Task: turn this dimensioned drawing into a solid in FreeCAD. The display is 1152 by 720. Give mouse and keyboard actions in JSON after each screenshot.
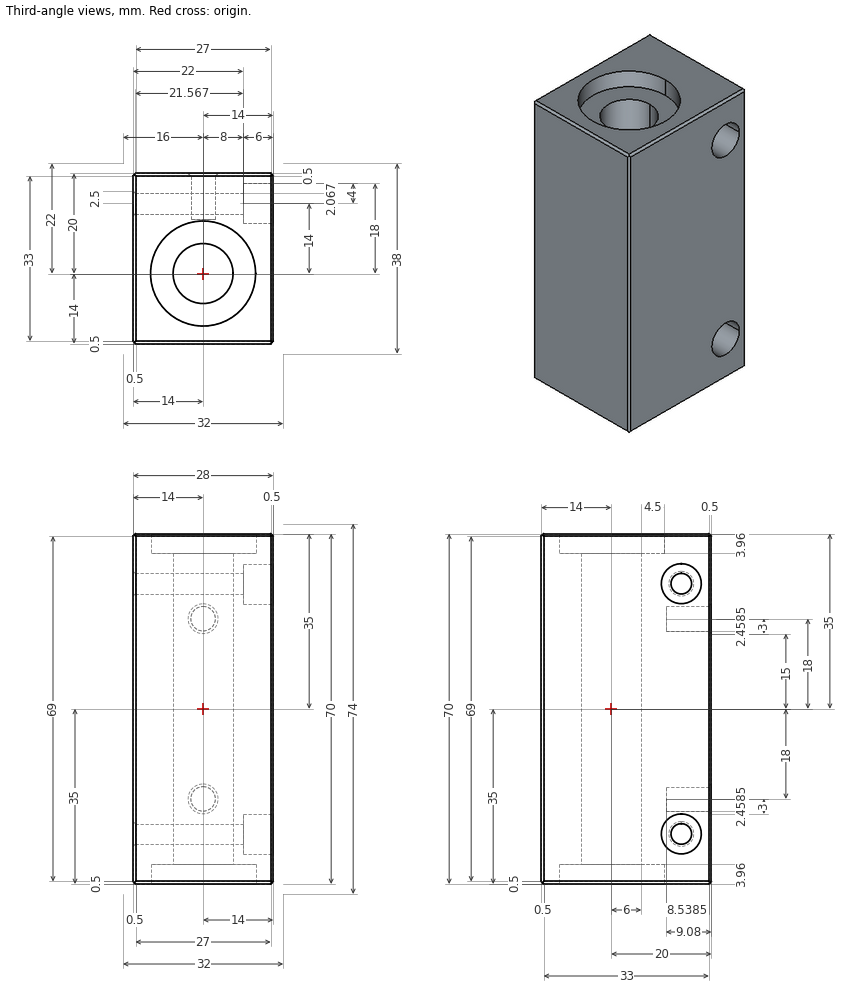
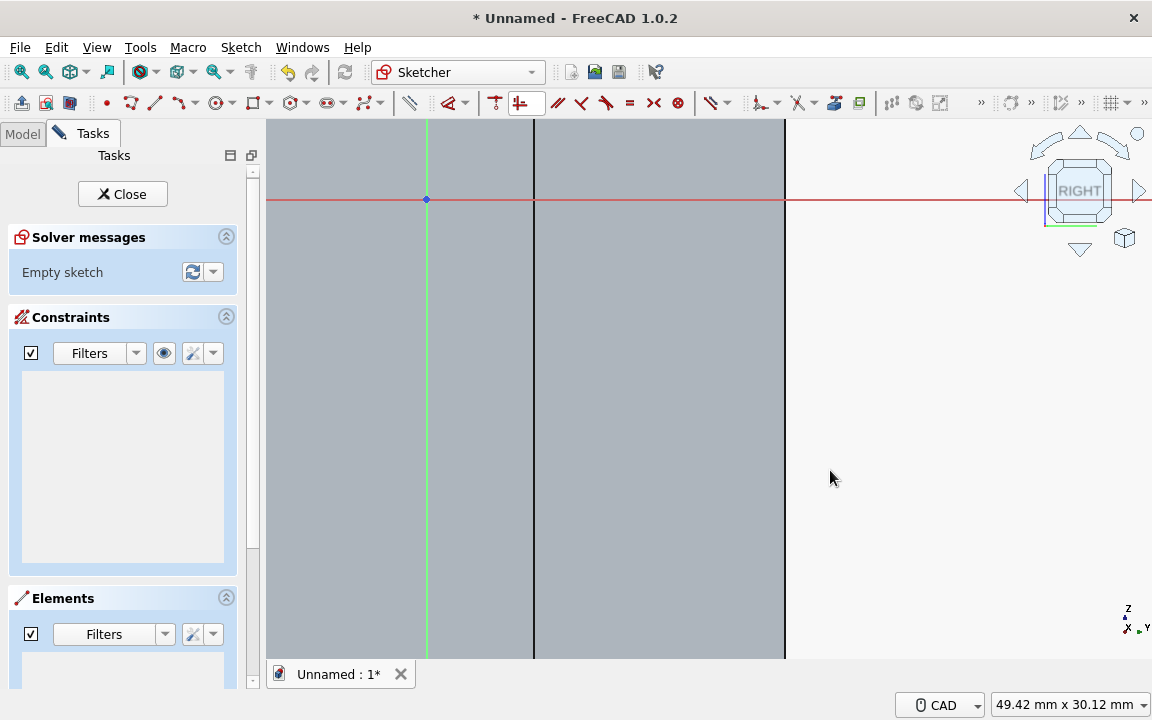
{"action": "left_click", "coordinate": [132, 104]}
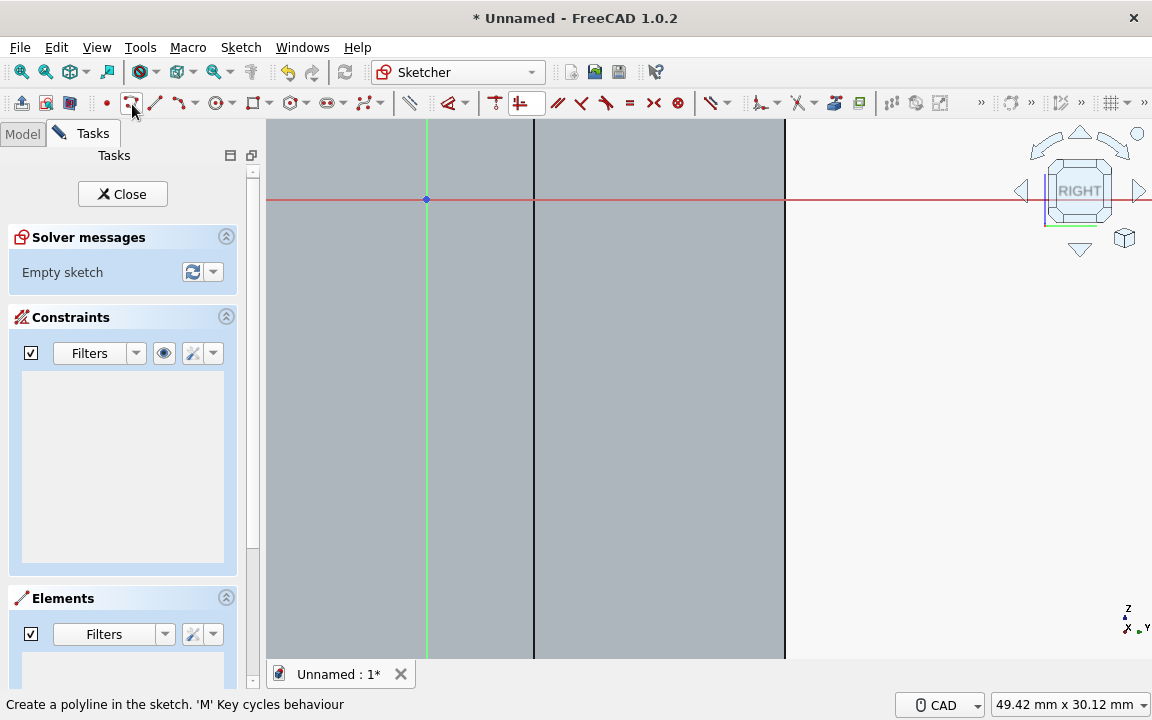
{"action": "left_click", "coordinate": [623, 522]}
{"action": "left_click", "coordinate": [623, 566]}
{"action": "left_click", "coordinate": [776, 566]}
{"action": "left_click", "coordinate": [785, 576]}
{"action": "left_click", "coordinate": [785, 522]}
{"action": "left_click", "coordinate": [623, 523]}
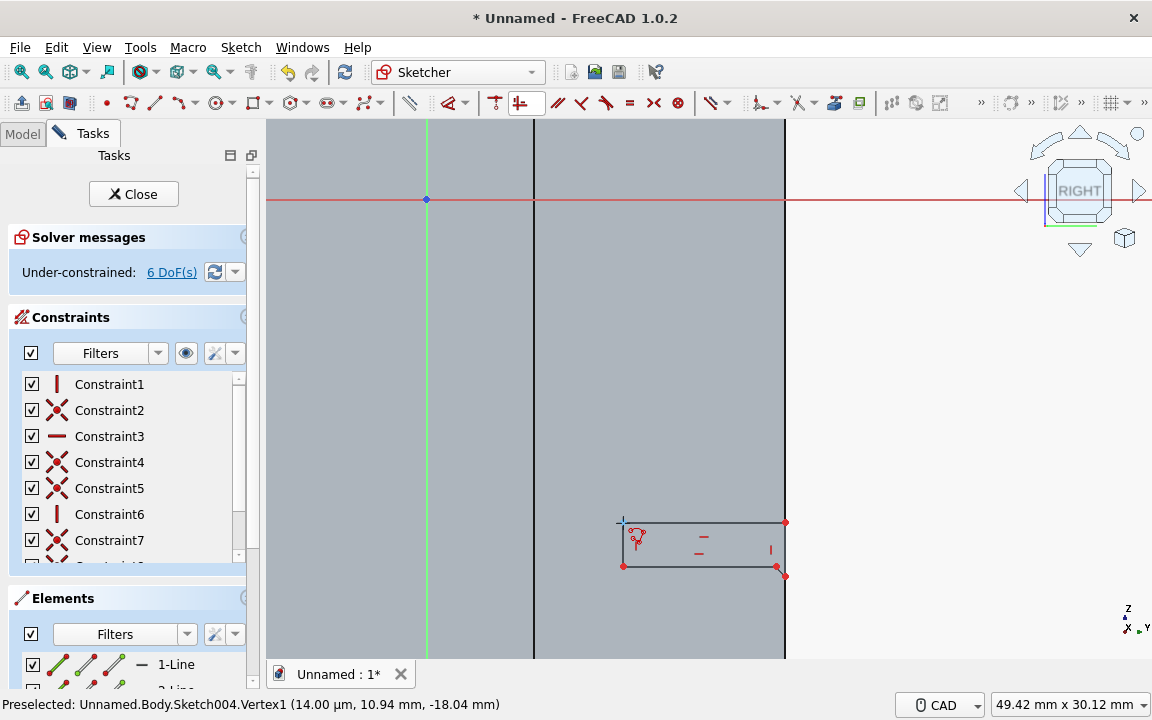
{"action": "left_click", "coordinate": [156, 104]}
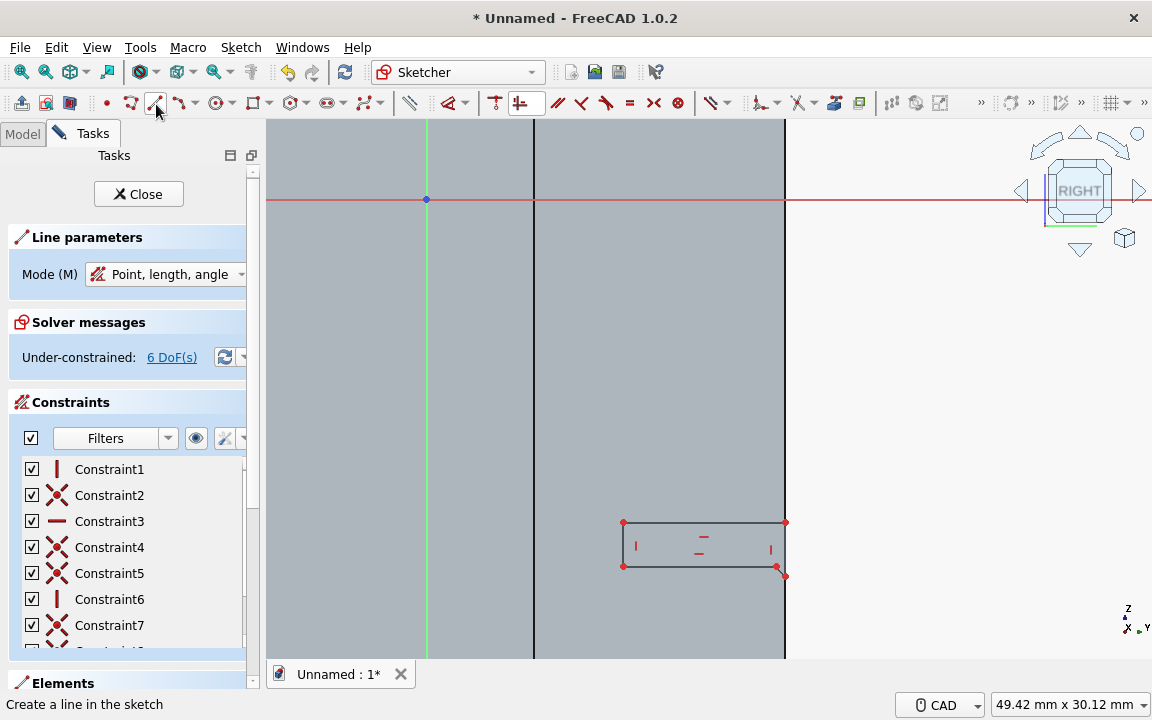
{"action": "left_click", "coordinate": [802, 522]}
{"action": "left_click", "coordinate": [850, 522]}
{"action": "key", "text": "Escape"}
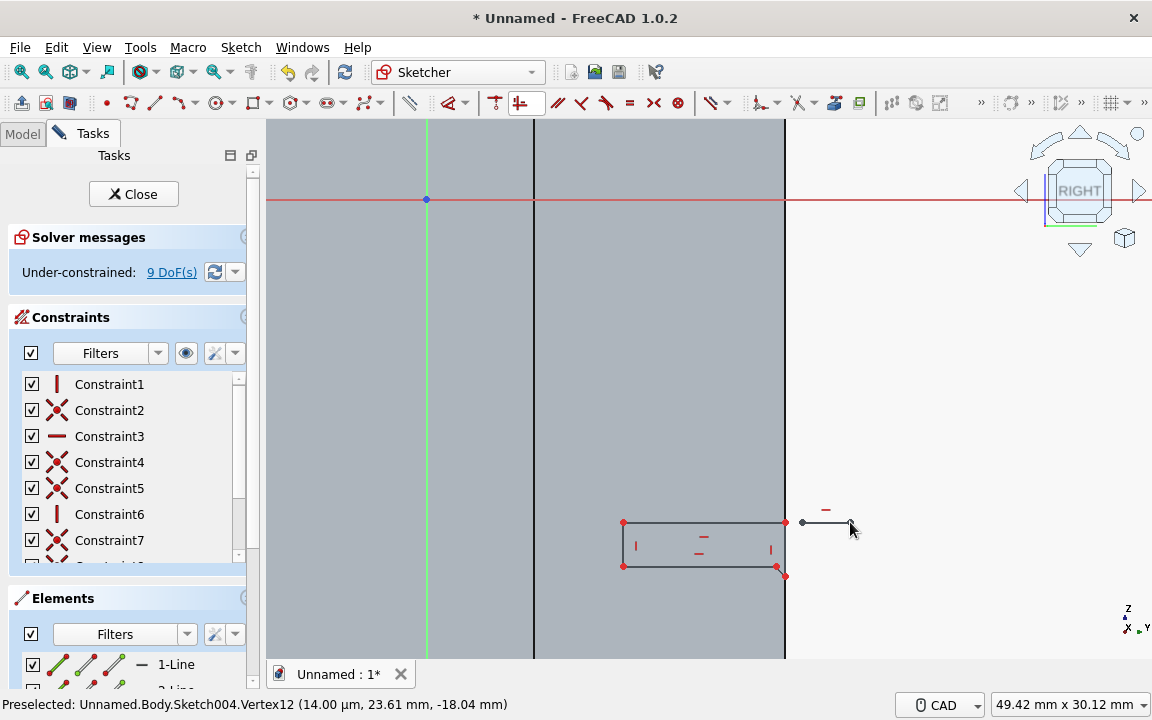
{"action": "left_click", "coordinate": [816, 523]}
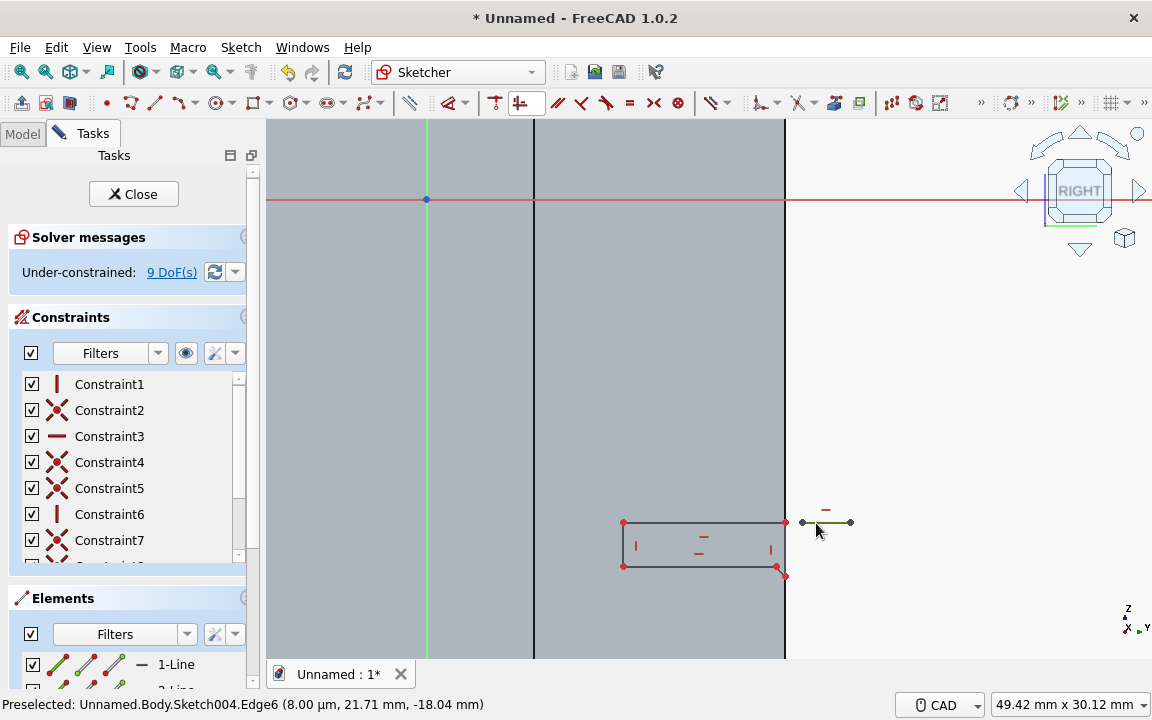
{"action": "left_click", "coordinate": [410, 104]}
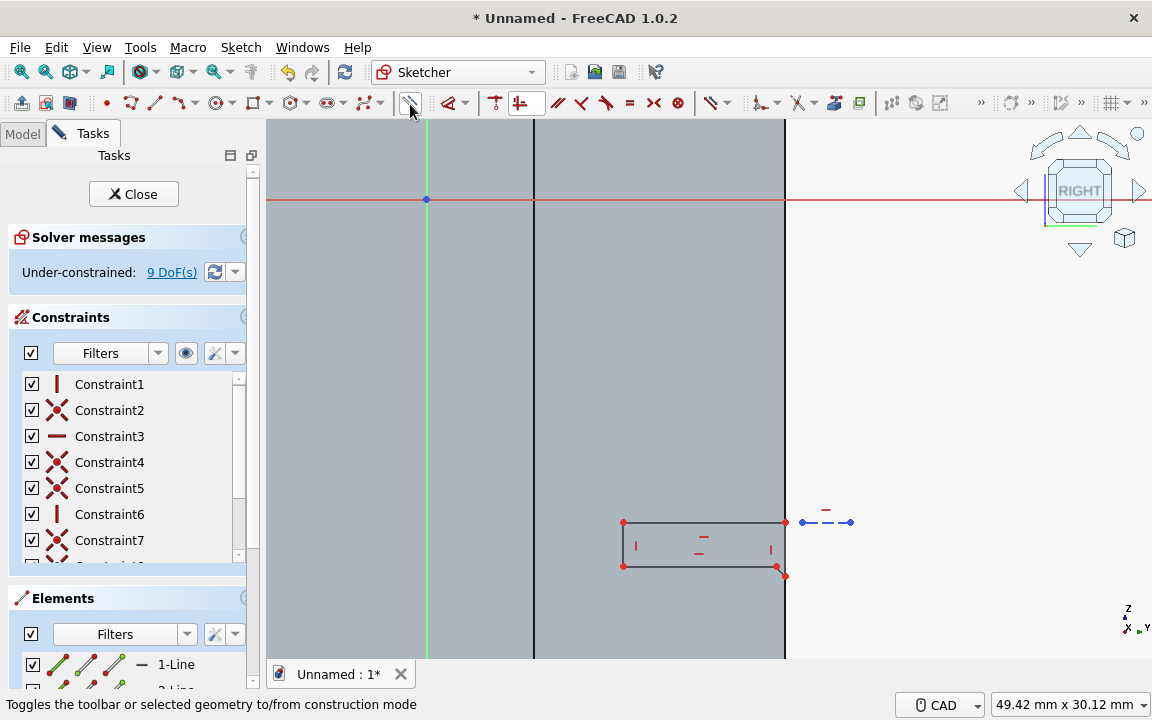
{"action": "left_click", "coordinate": [448, 104]}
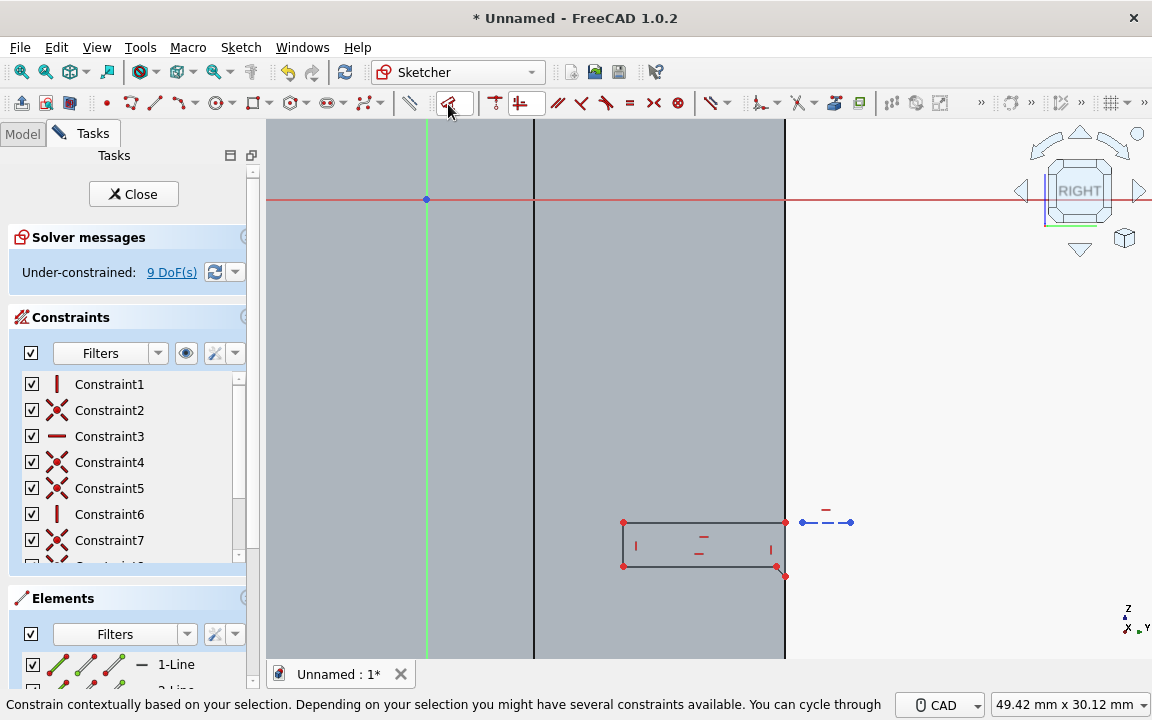
{"action": "scroll", "coordinate": [785, 561], "scroll_direction": "up", "scroll_amount": 2}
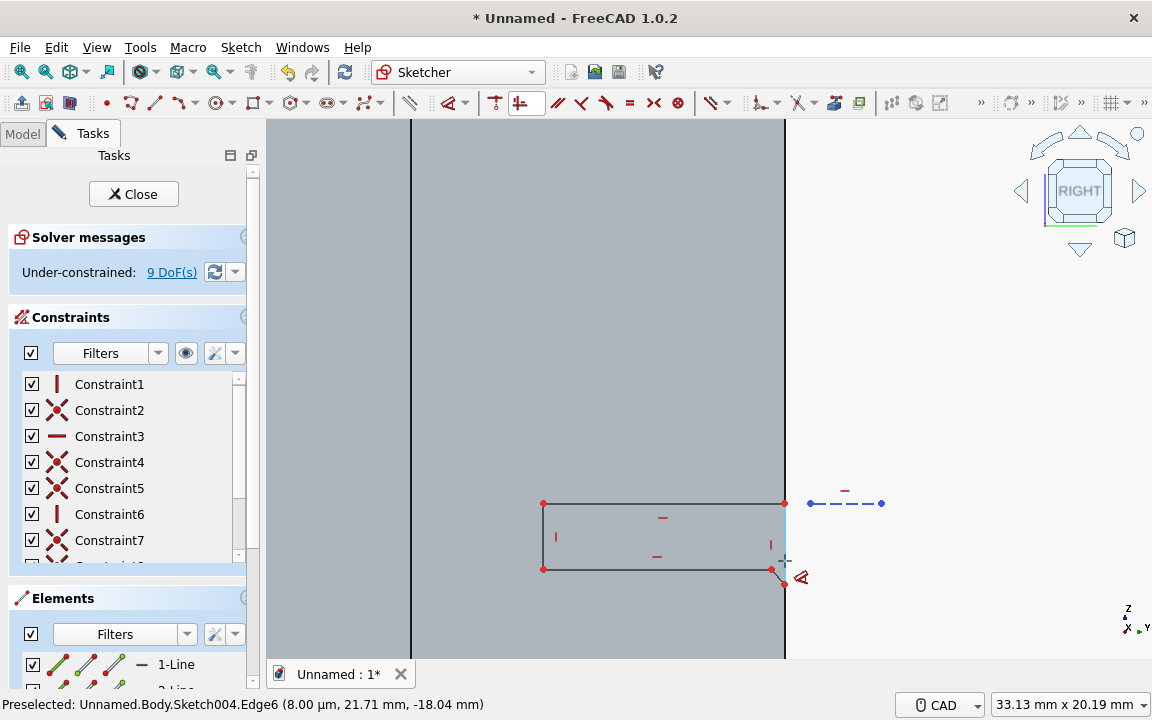
{"action": "left_click", "coordinate": [785, 560]}
{"action": "left_click", "coordinate": [819, 544]}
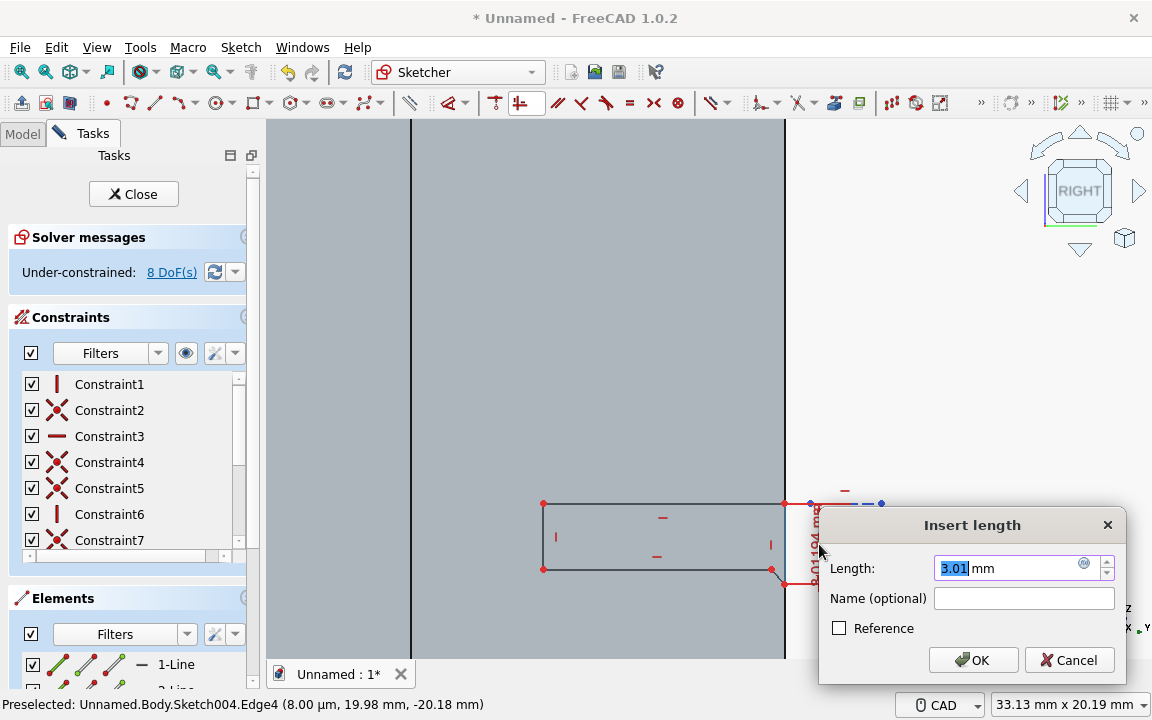
{"action": "type", "text": "3"}
{"action": "key", "text": "Return"}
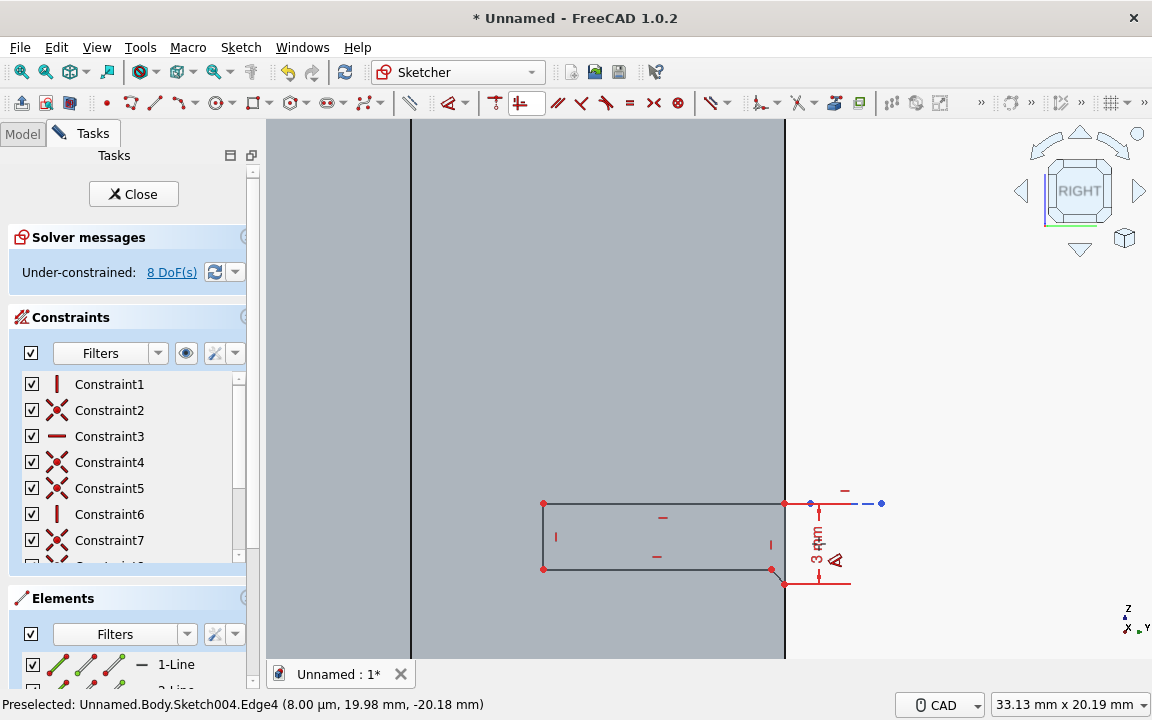
{"action": "left_click", "coordinate": [543, 504]}
{"action": "left_click", "coordinate": [577, 325]}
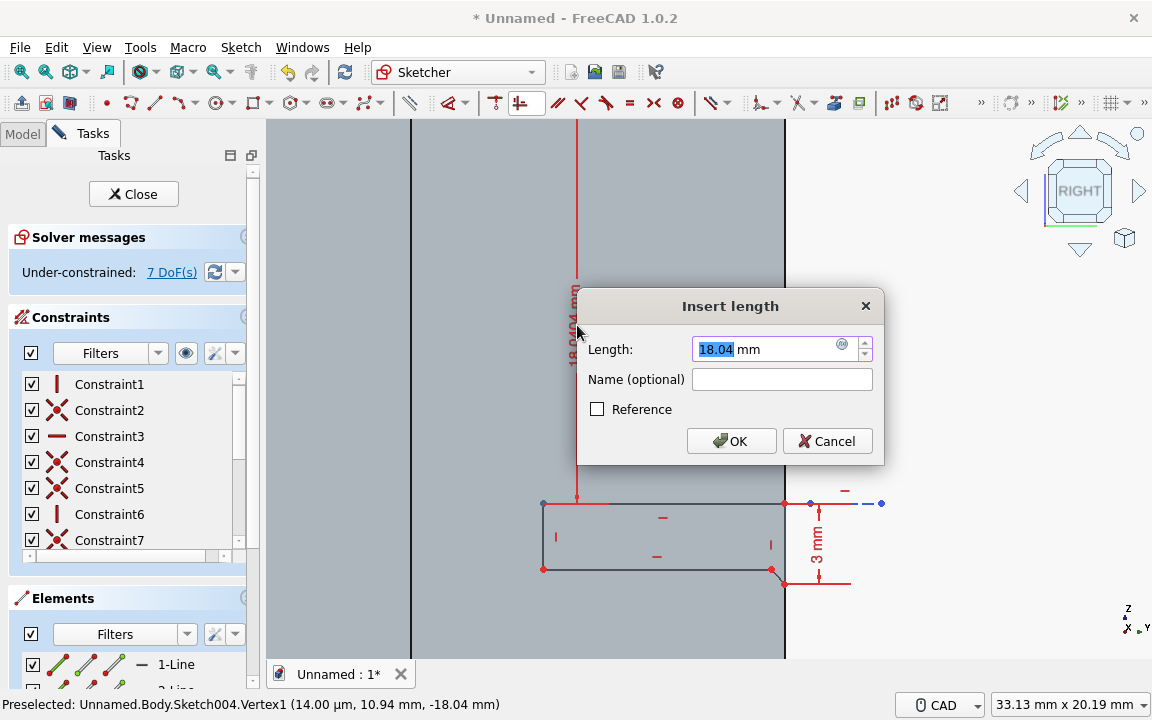
{"action": "type", "text": "18"}
{"action": "key", "text": "Return"}